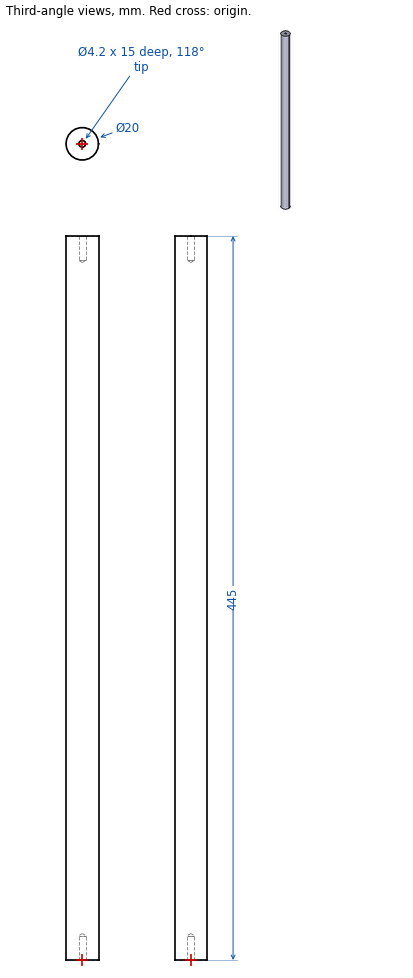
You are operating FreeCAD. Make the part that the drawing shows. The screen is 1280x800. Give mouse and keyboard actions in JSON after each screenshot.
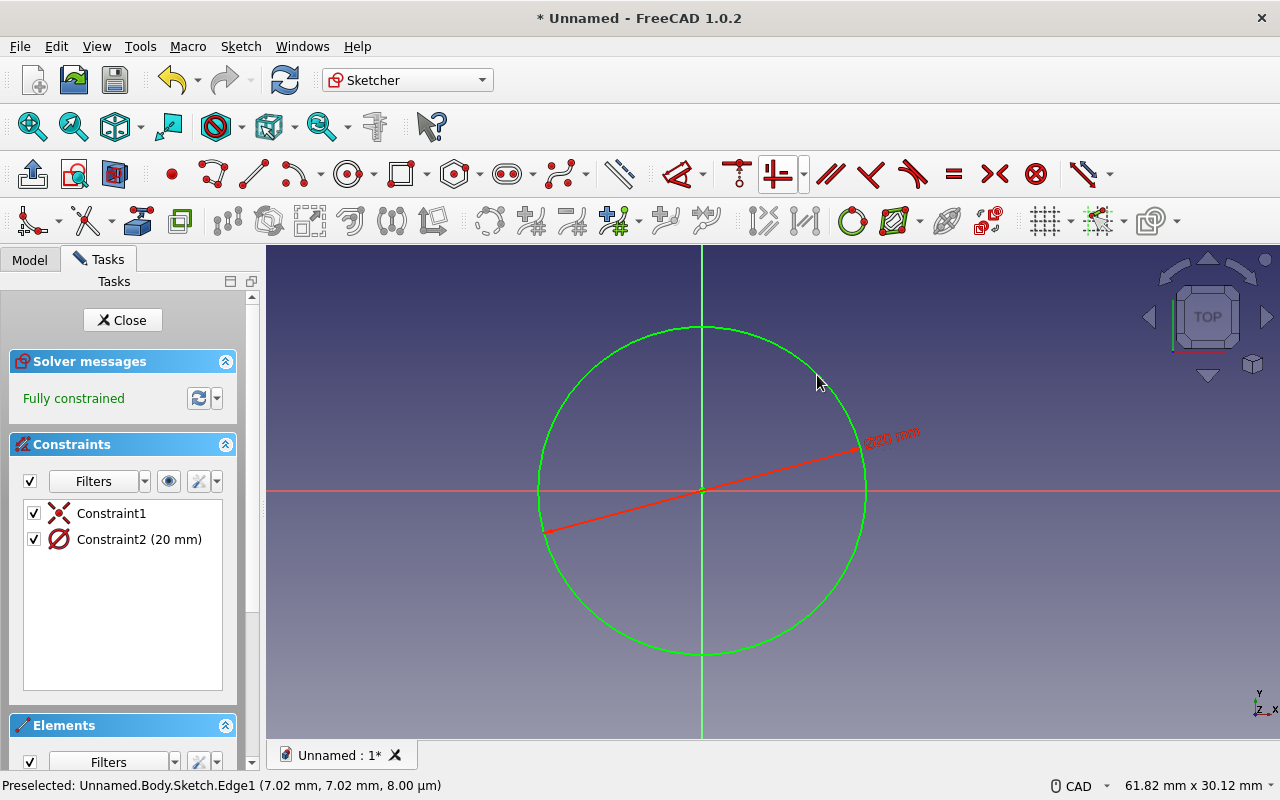
{"action": "left_click", "coordinate": [123, 320]}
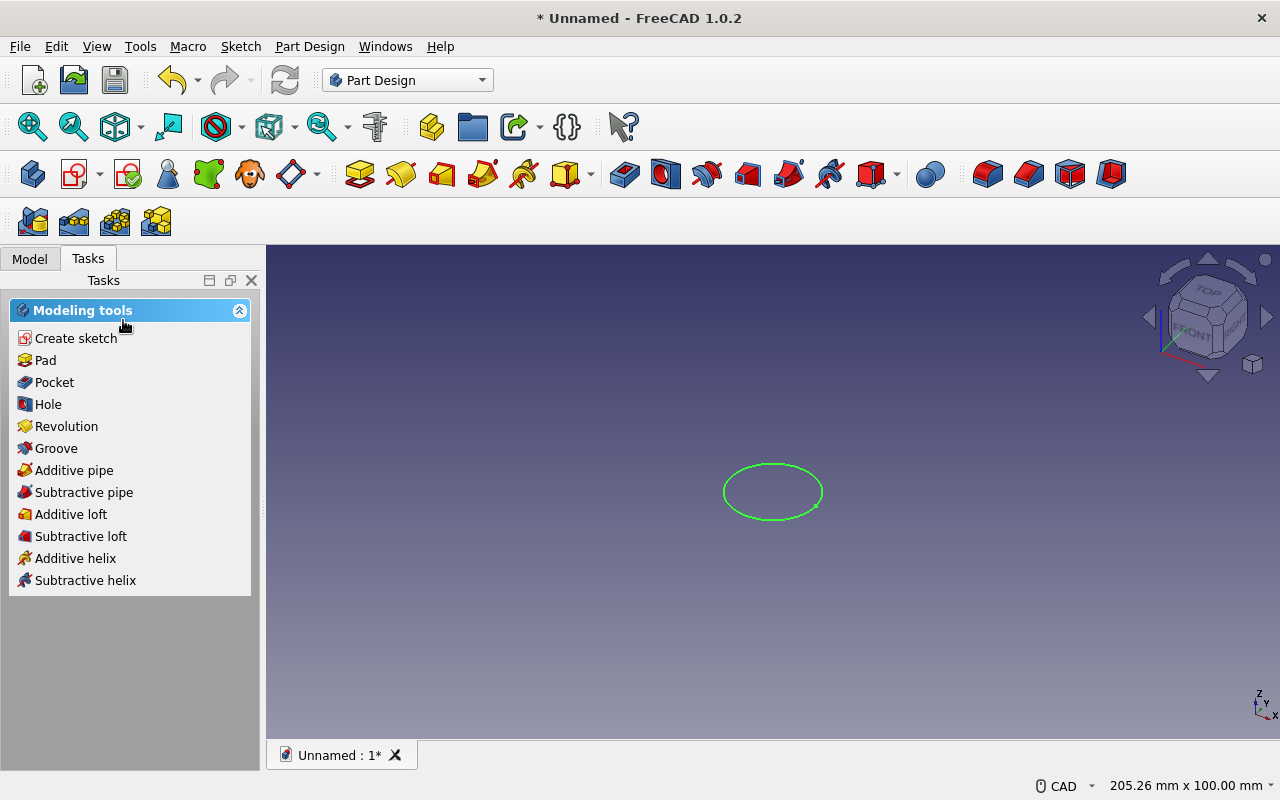
{"action": "left_click", "coordinate": [360, 174]}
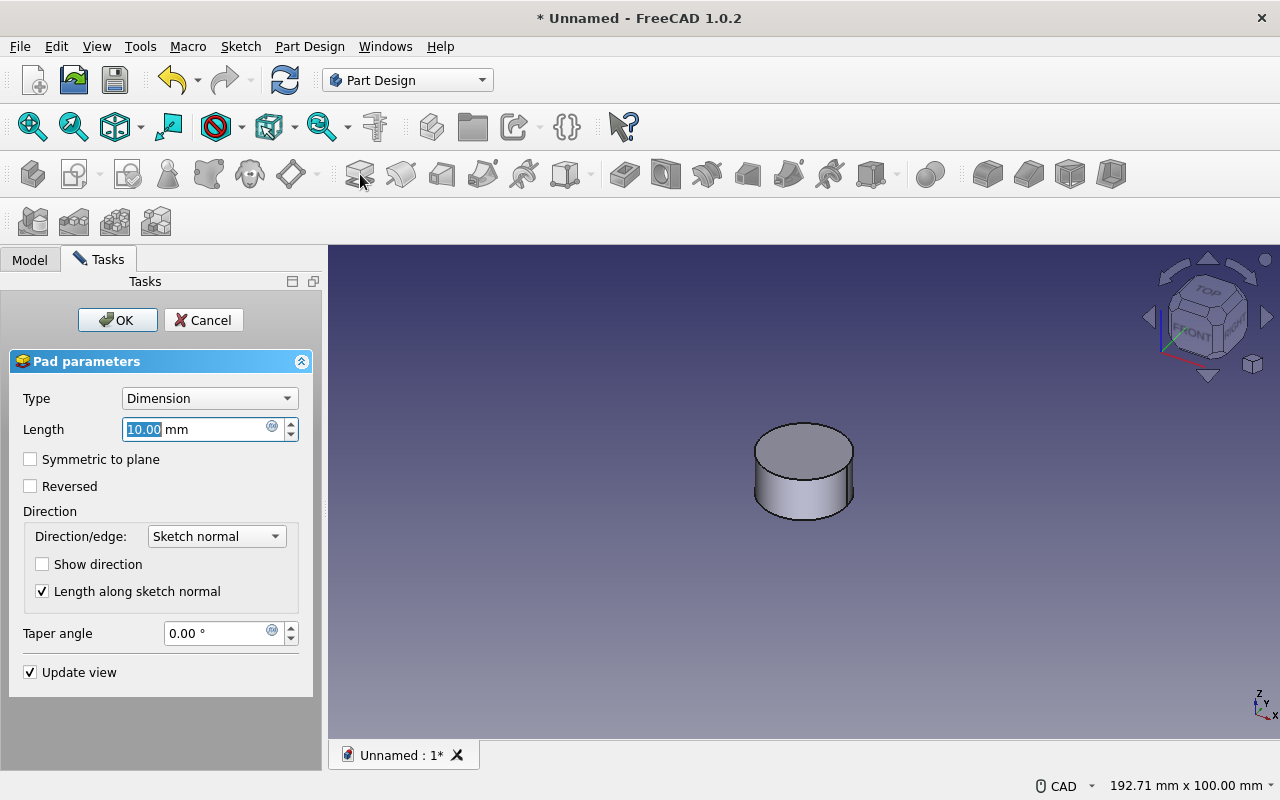
{"action": "type", "text": "445"}
{"action": "key", "text": "Tab"}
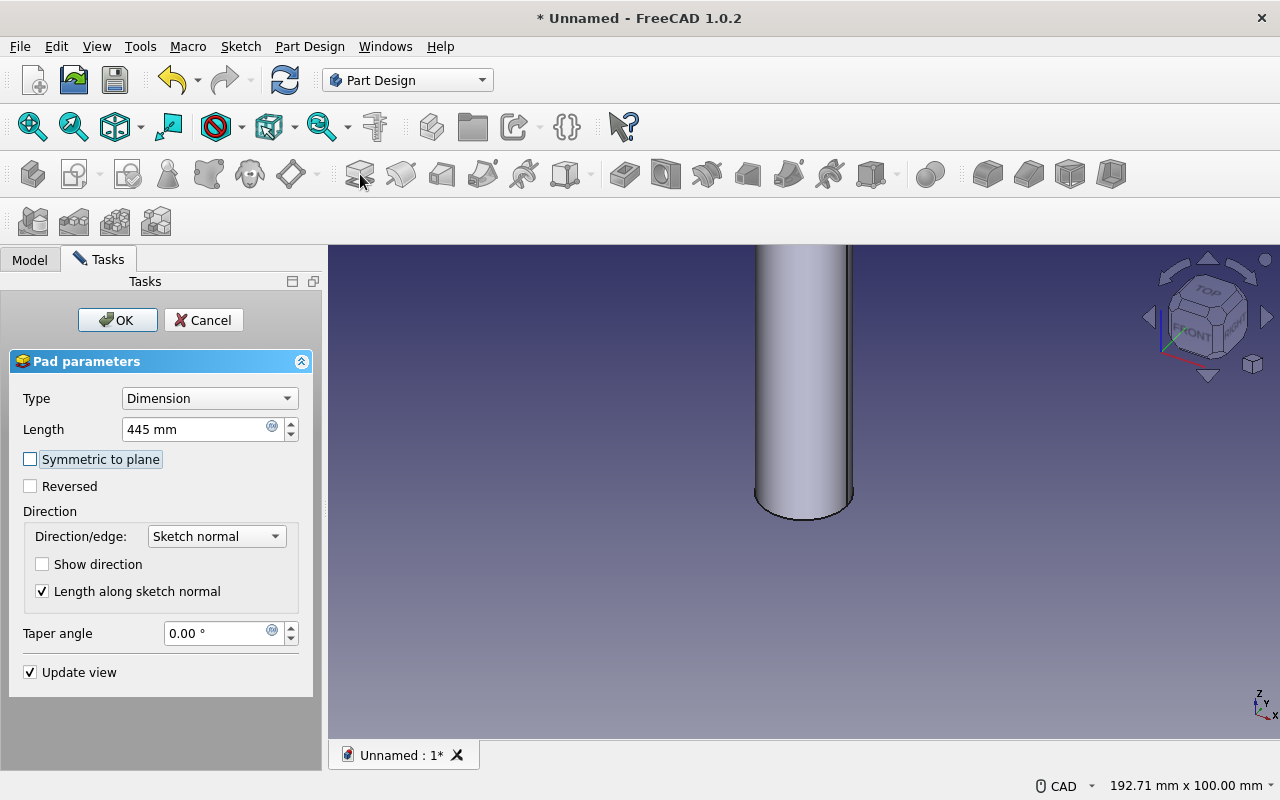
{"action": "left_click", "coordinate": [118, 320]}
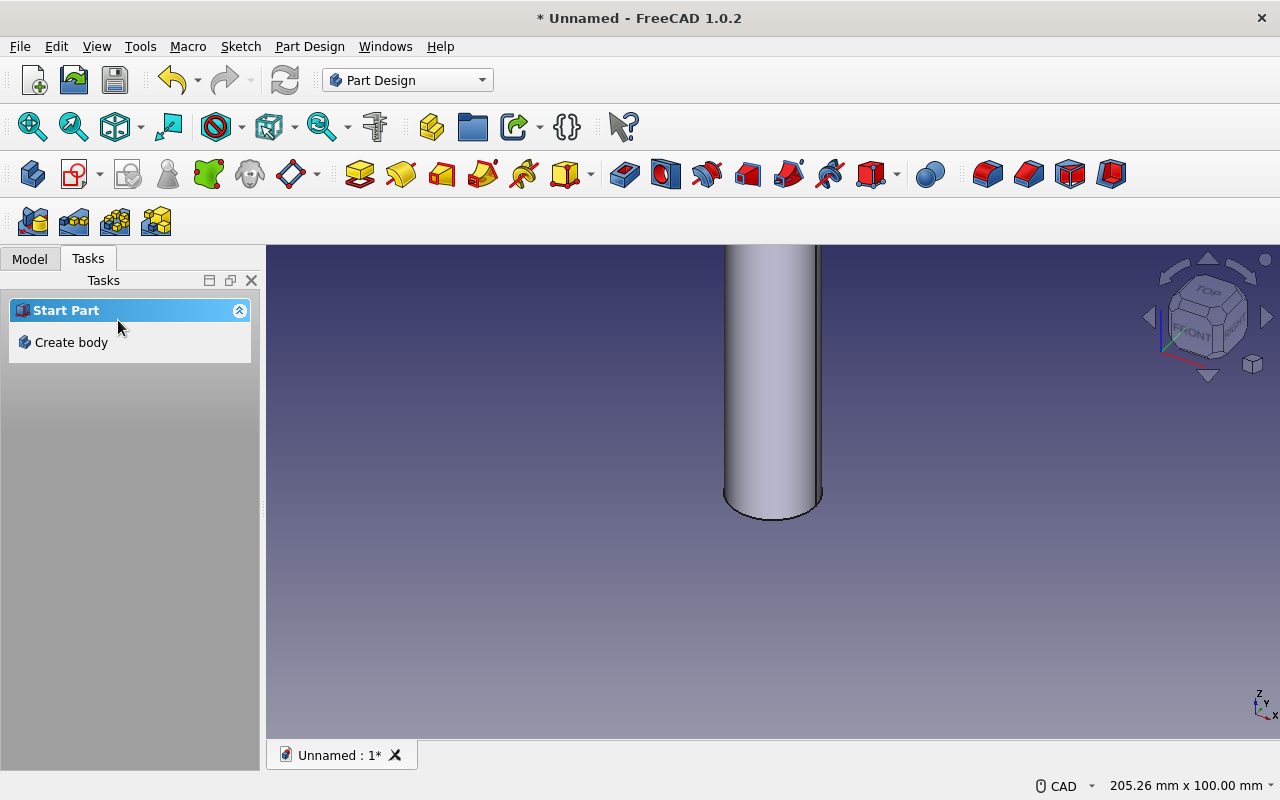
{"action": "key", "text": "v f"}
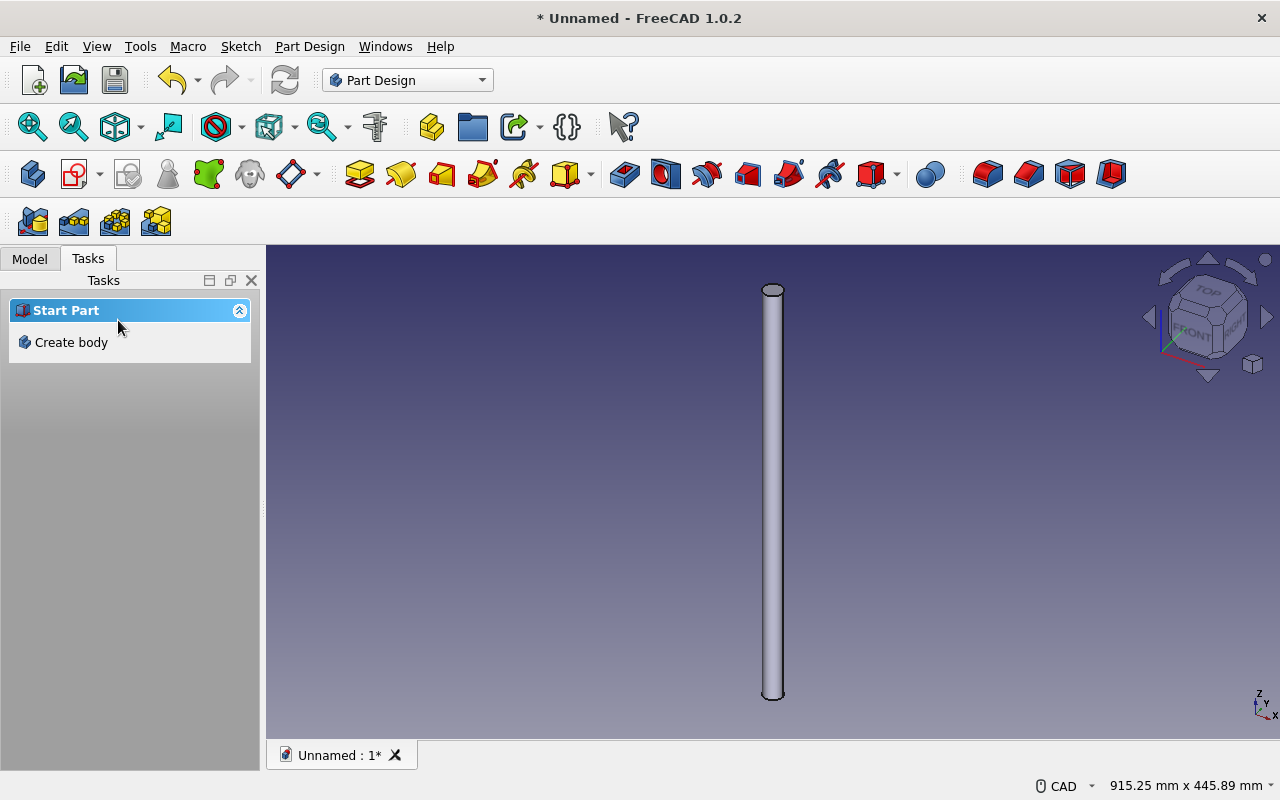
{"action": "key", "text": "0"}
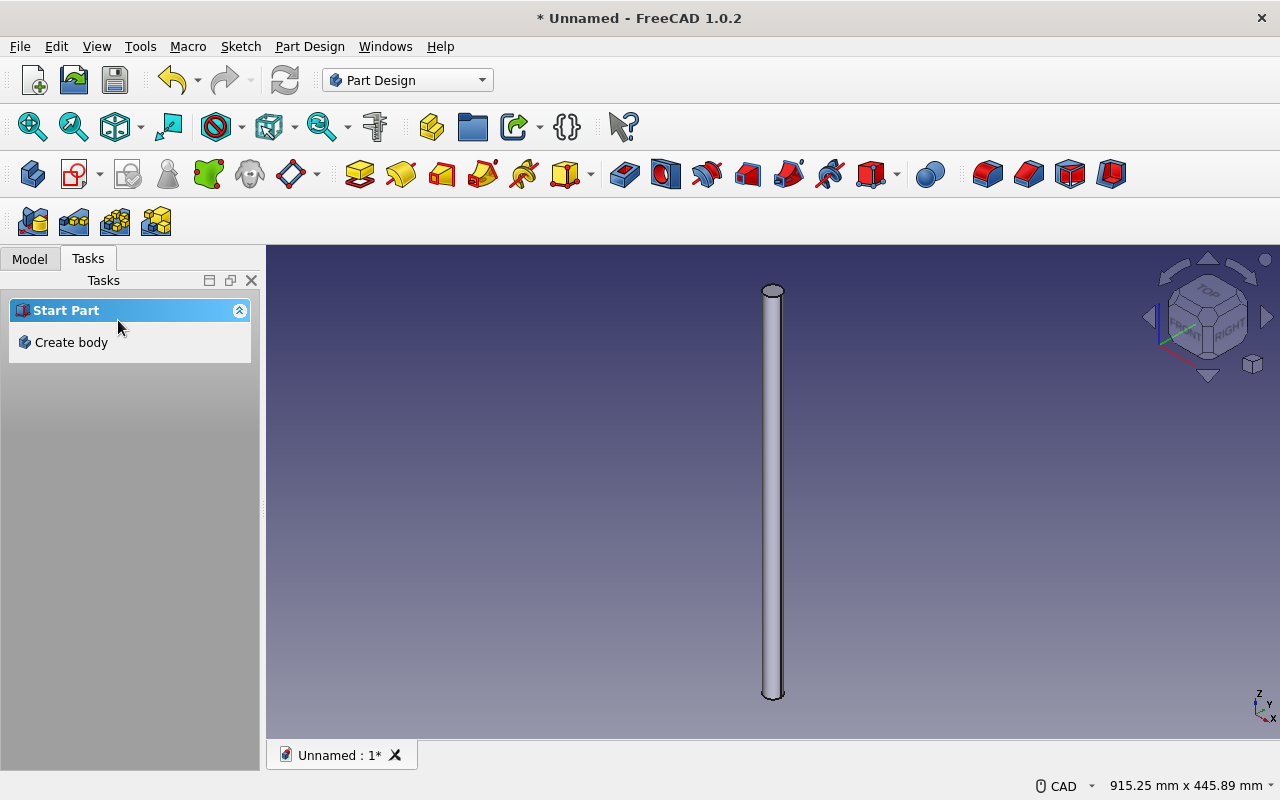
{"action": "key", "text": "2"}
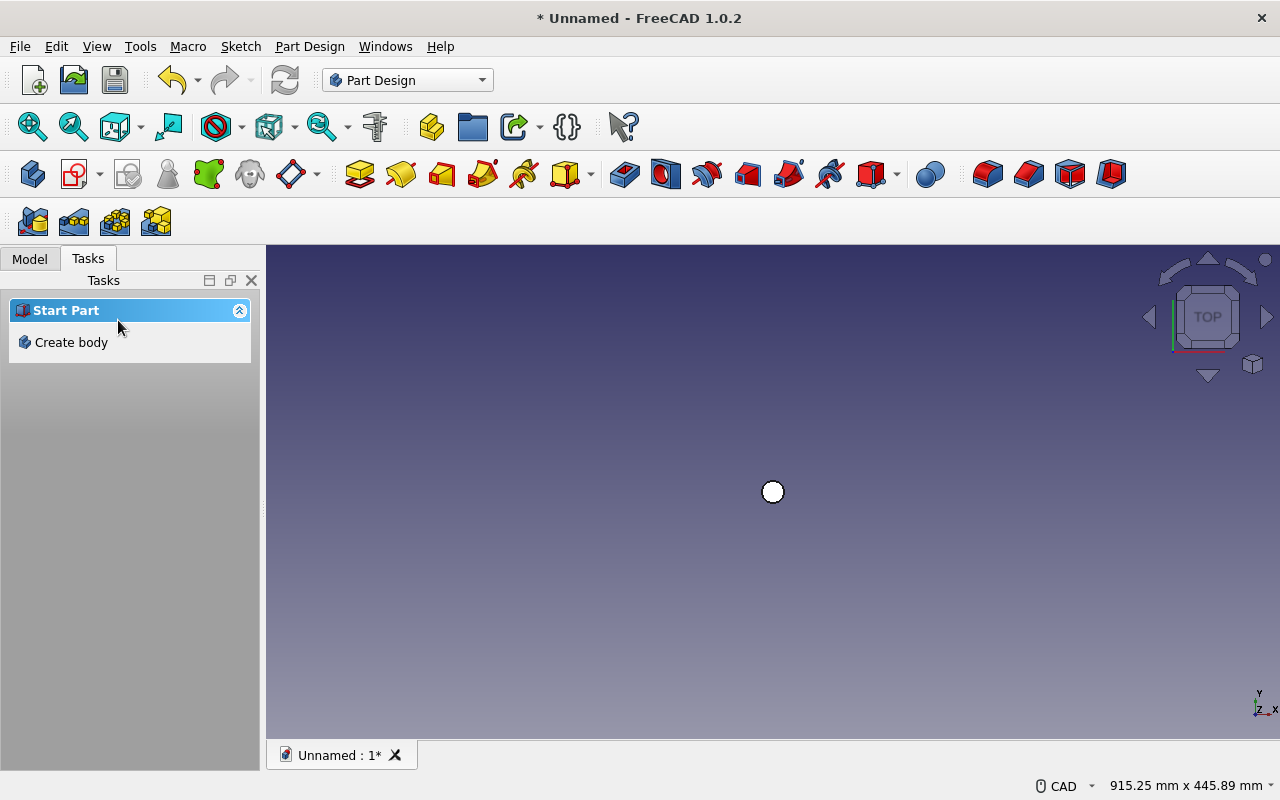
{"action": "key", "text": "v f"}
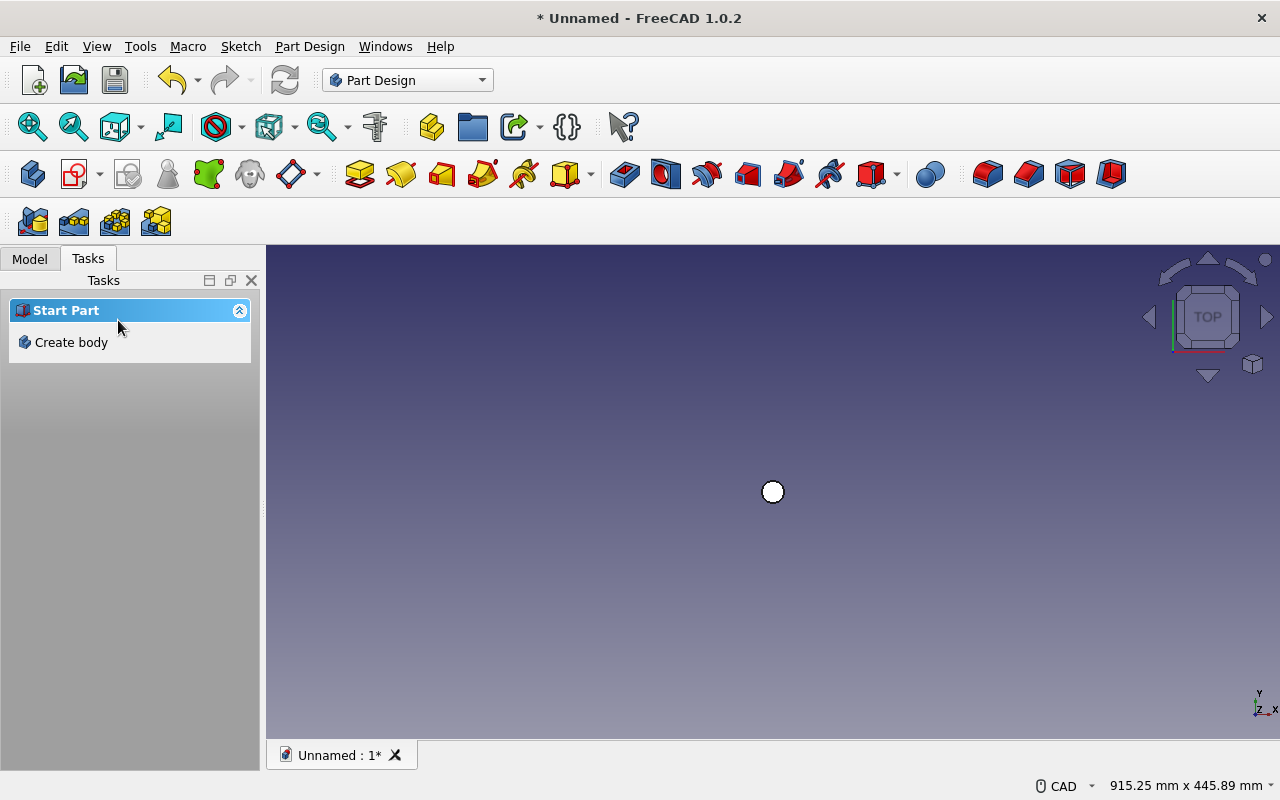
{"action": "left_click", "coordinate": [773, 491]}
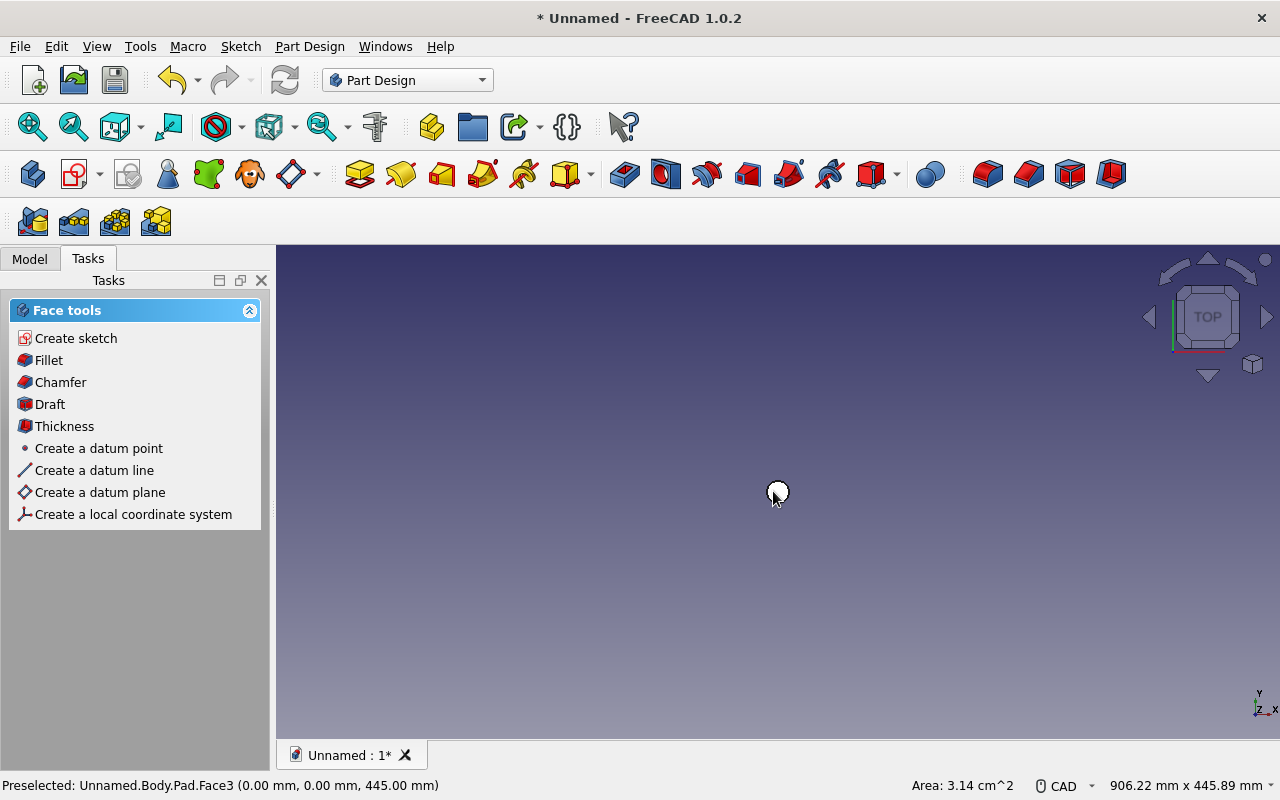
{"action": "left_click", "coordinate": [74, 174]}